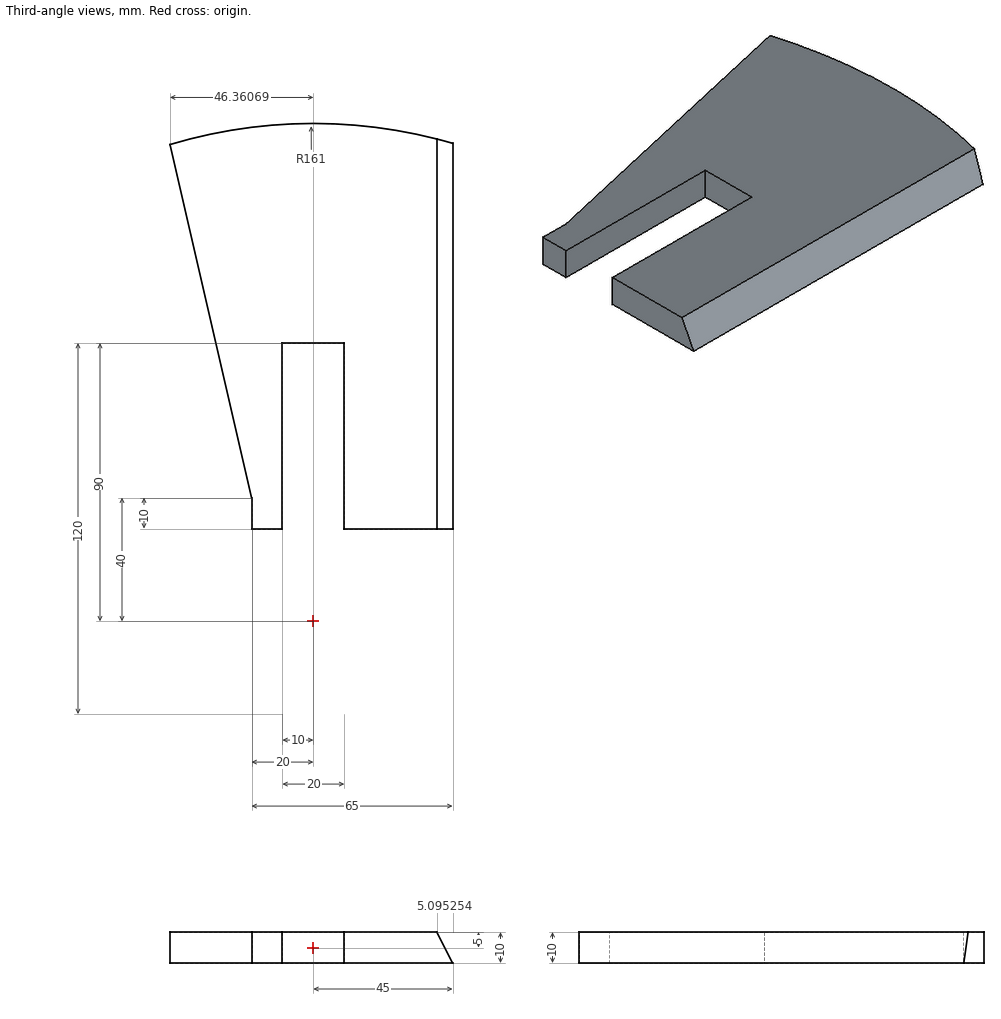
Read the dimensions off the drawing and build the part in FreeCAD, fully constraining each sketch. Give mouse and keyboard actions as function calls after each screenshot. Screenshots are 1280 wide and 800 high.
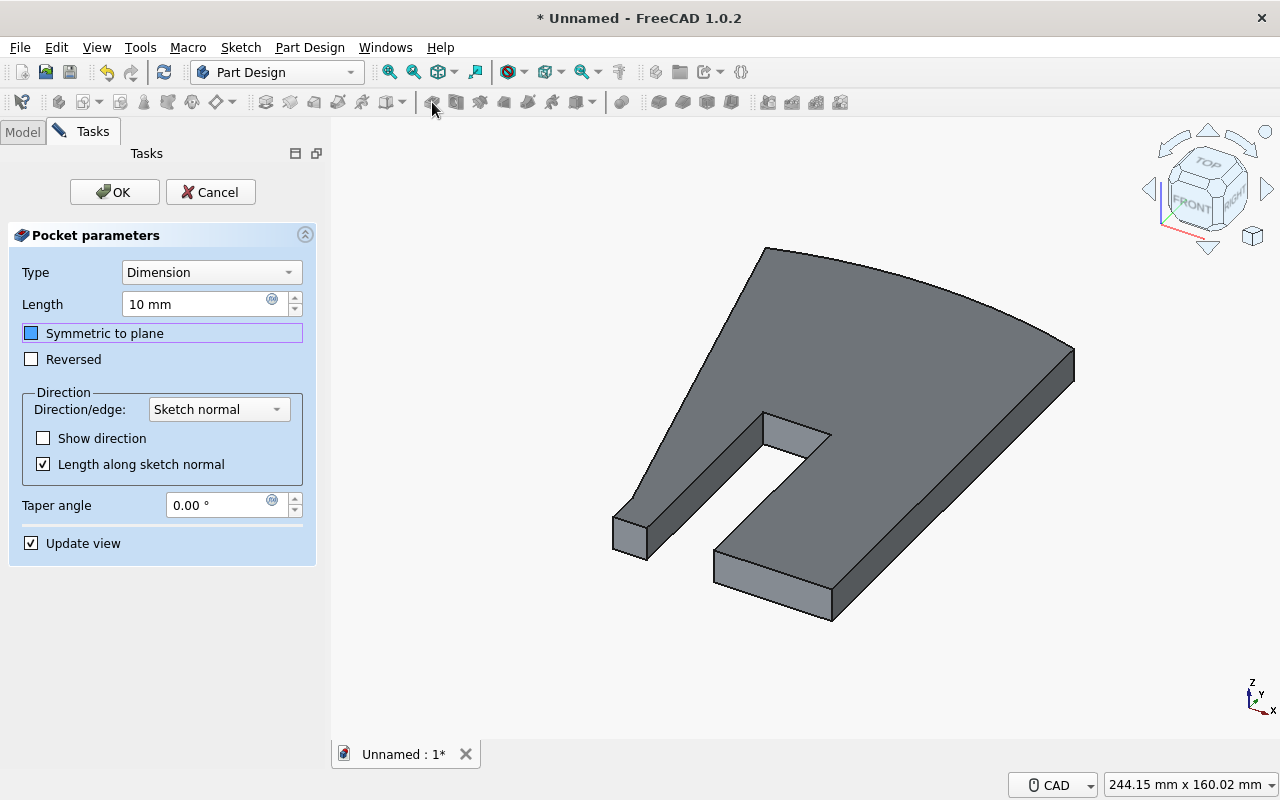
click(115, 192)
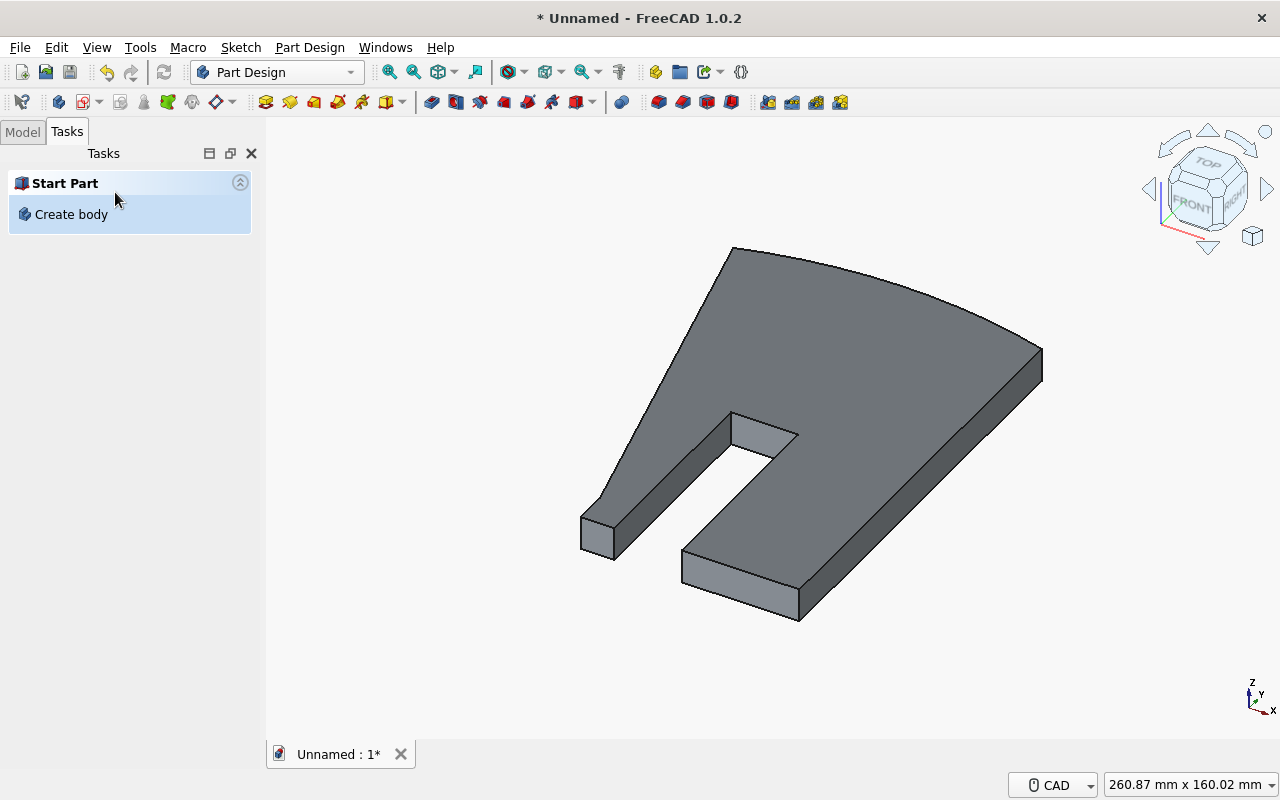
click(774, 596)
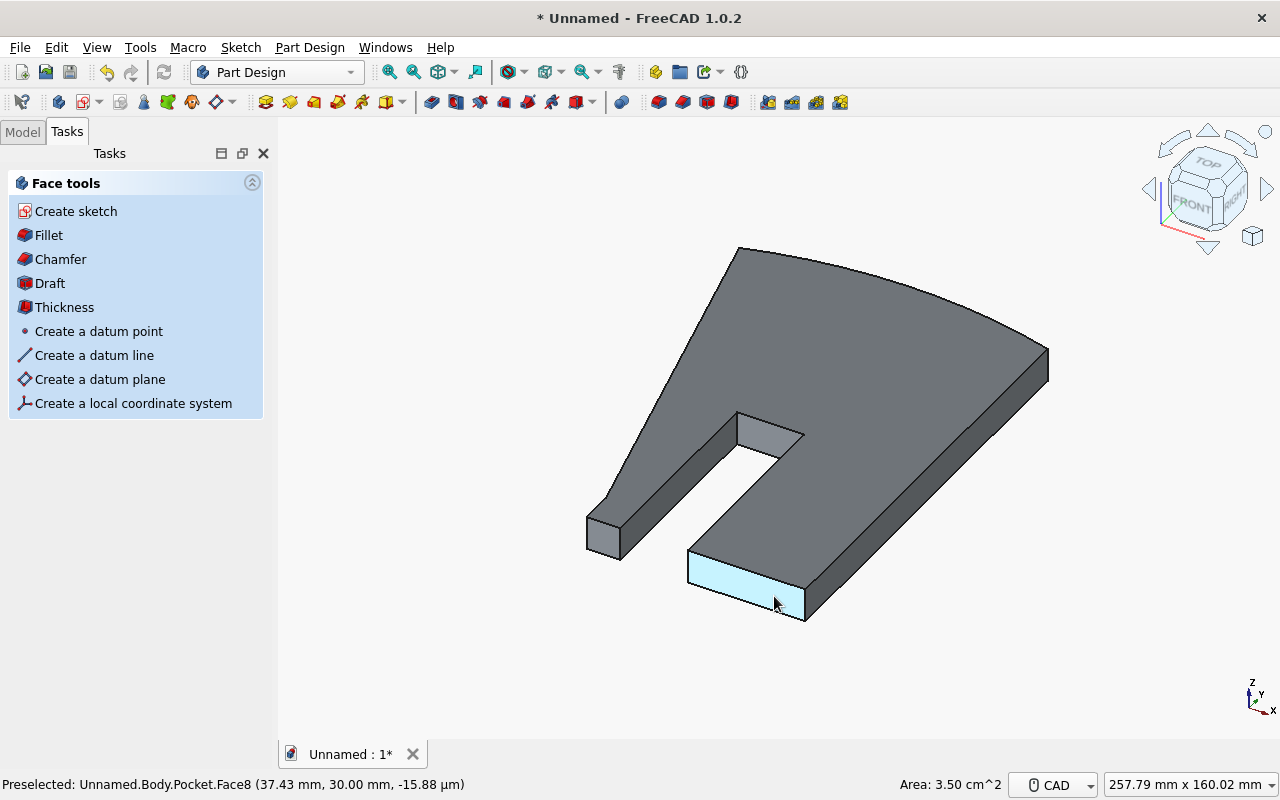
click(84, 102)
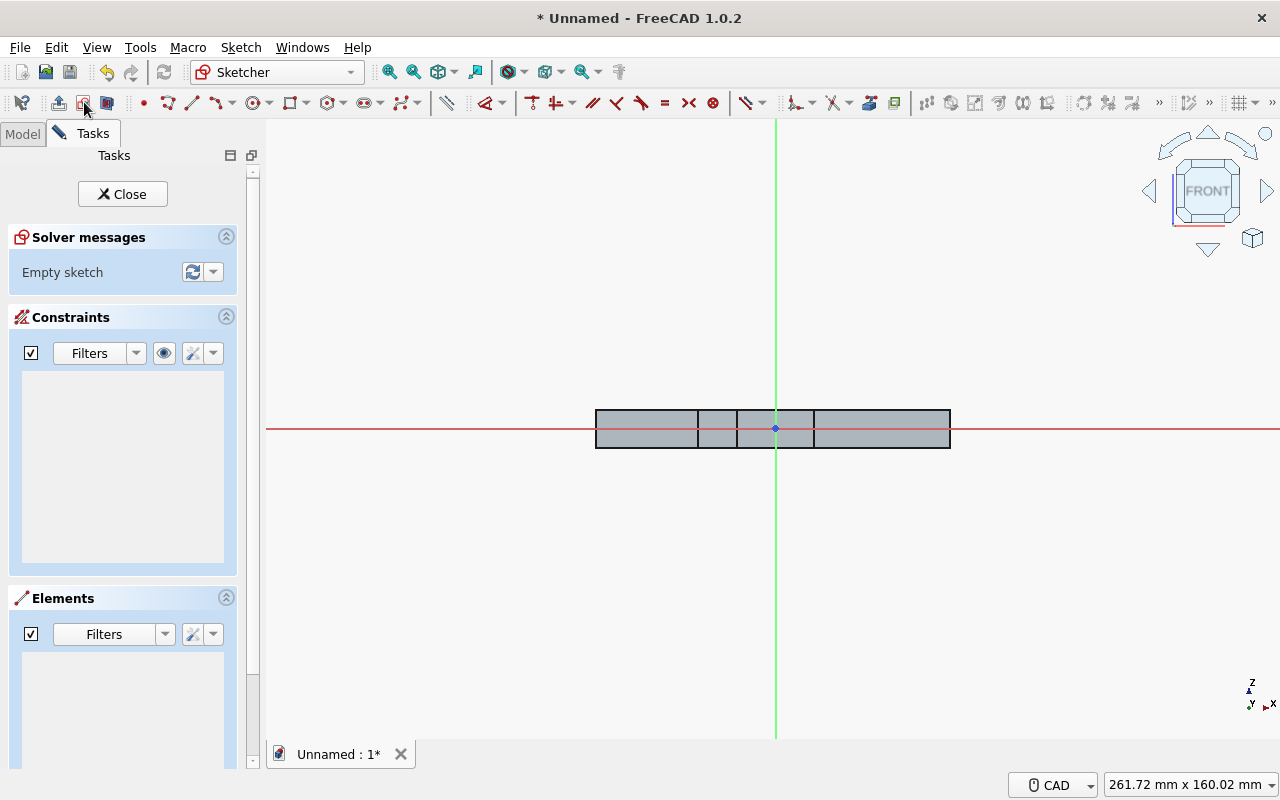
scroll(964, 429, up, 12)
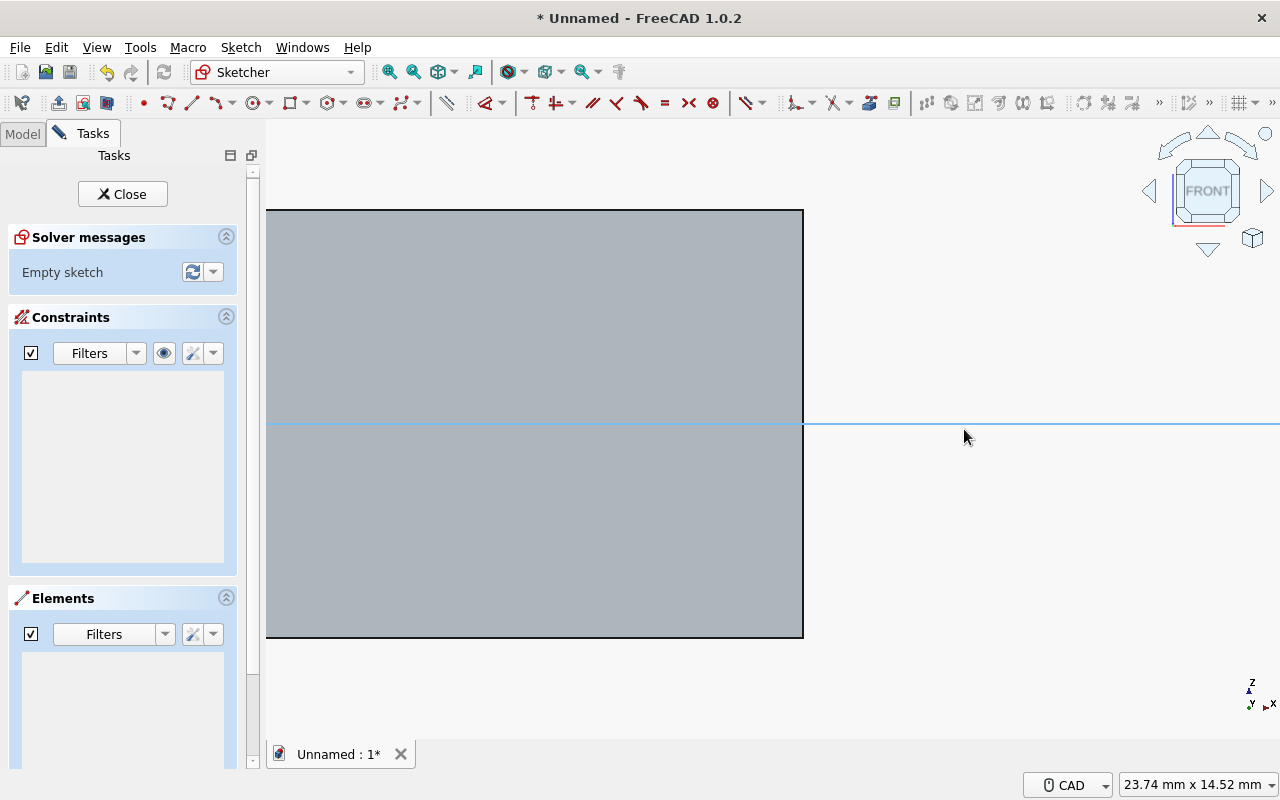
click(168, 104)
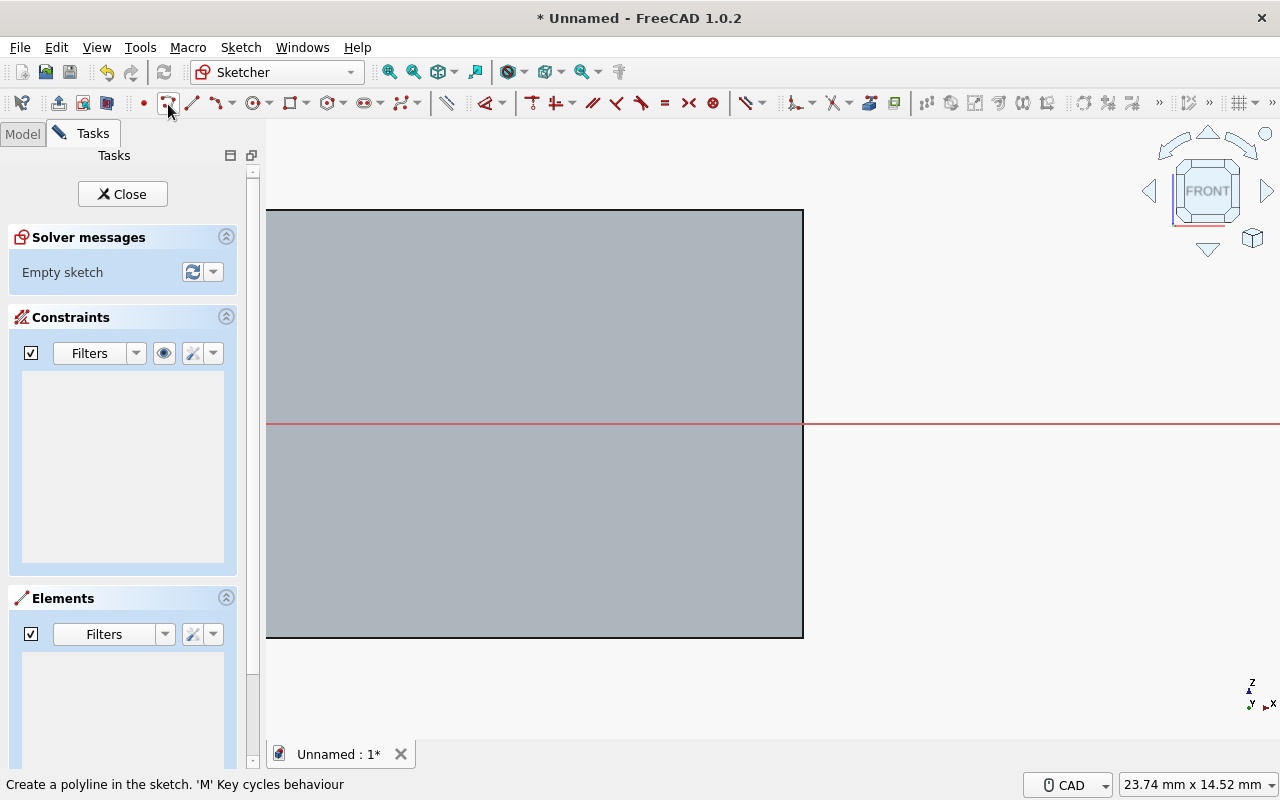
click(585, 210)
click(803, 638)
click(803, 210)
click(585, 211)
key(Escape)
key(Escape)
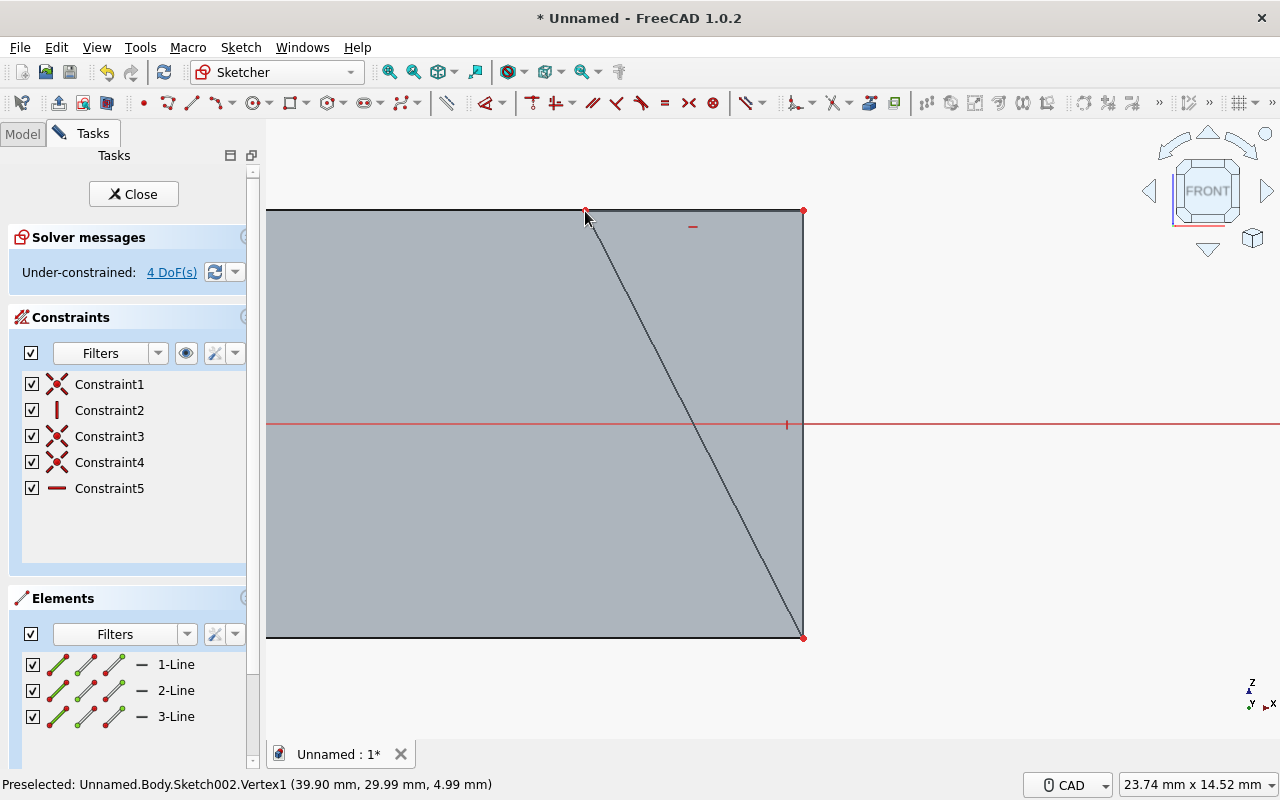
click(486, 104)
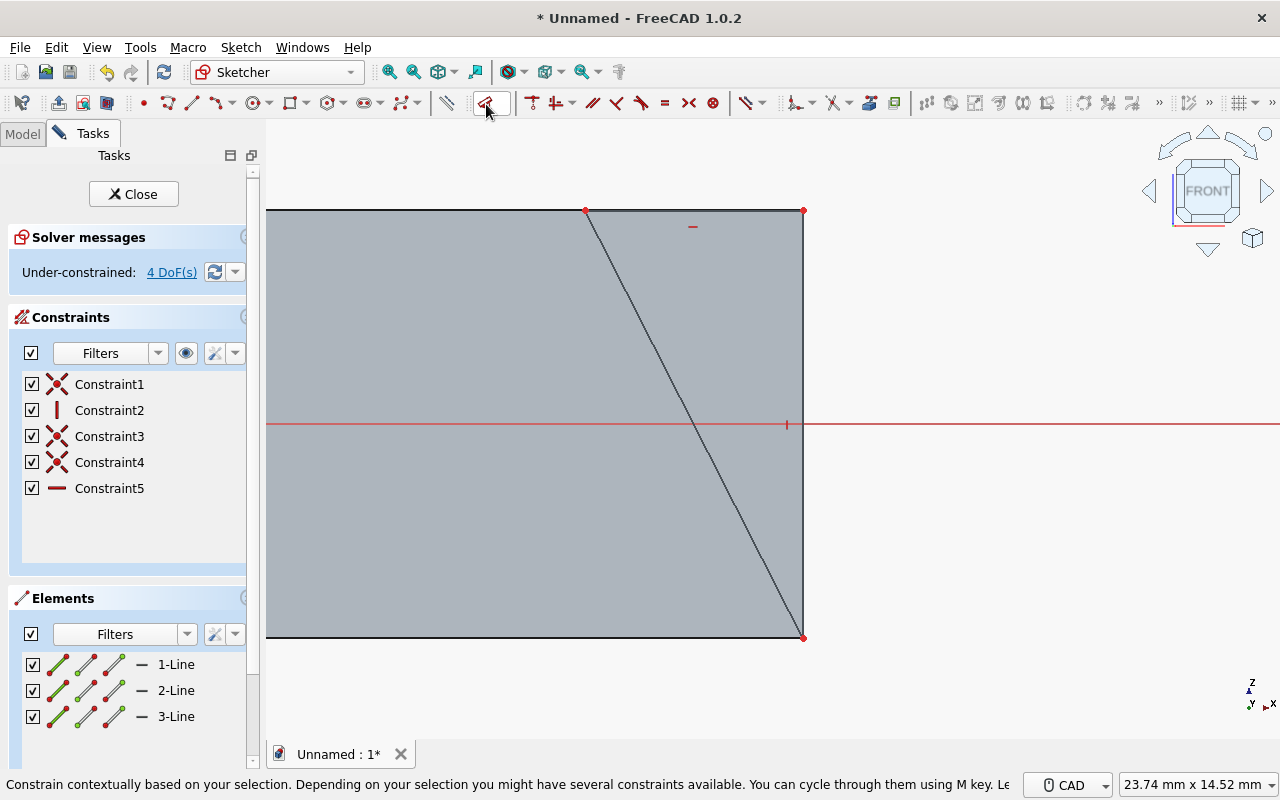
click(803, 511)
click(837, 327)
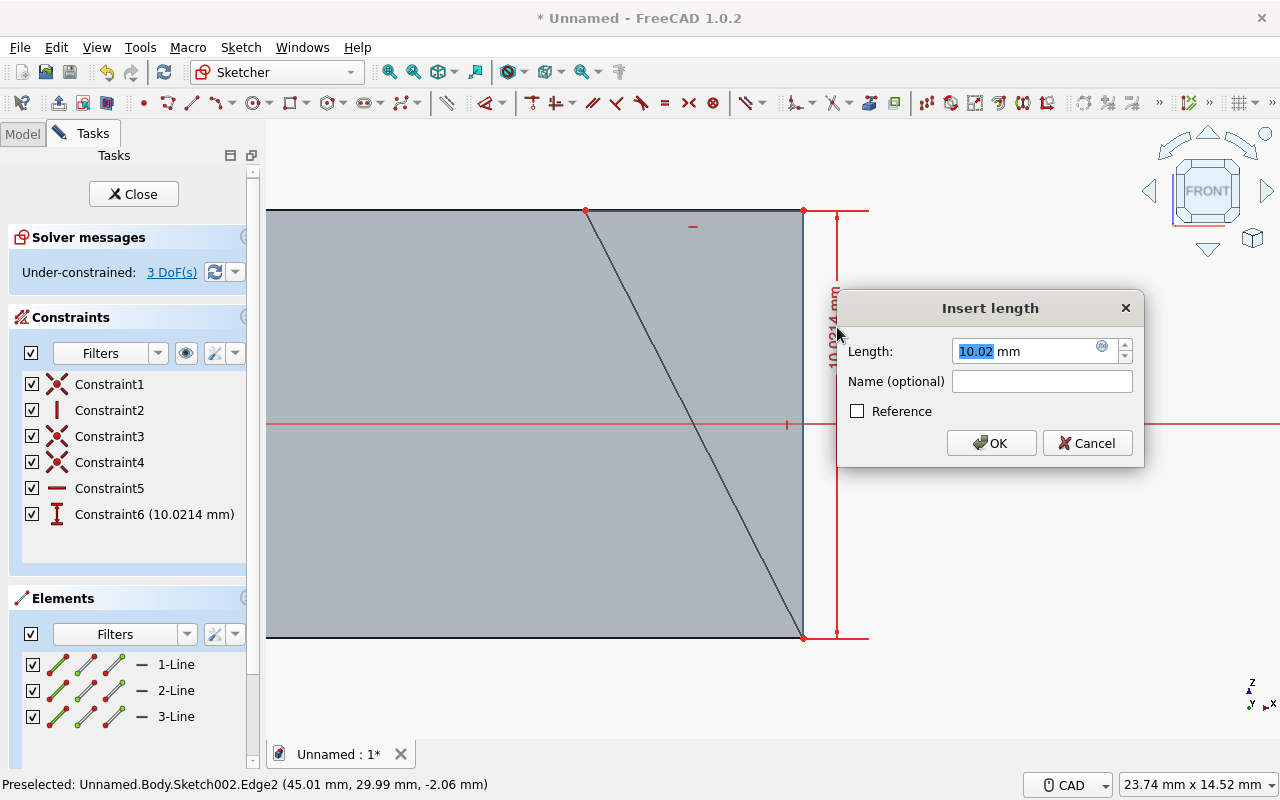
text(10)
key(Return)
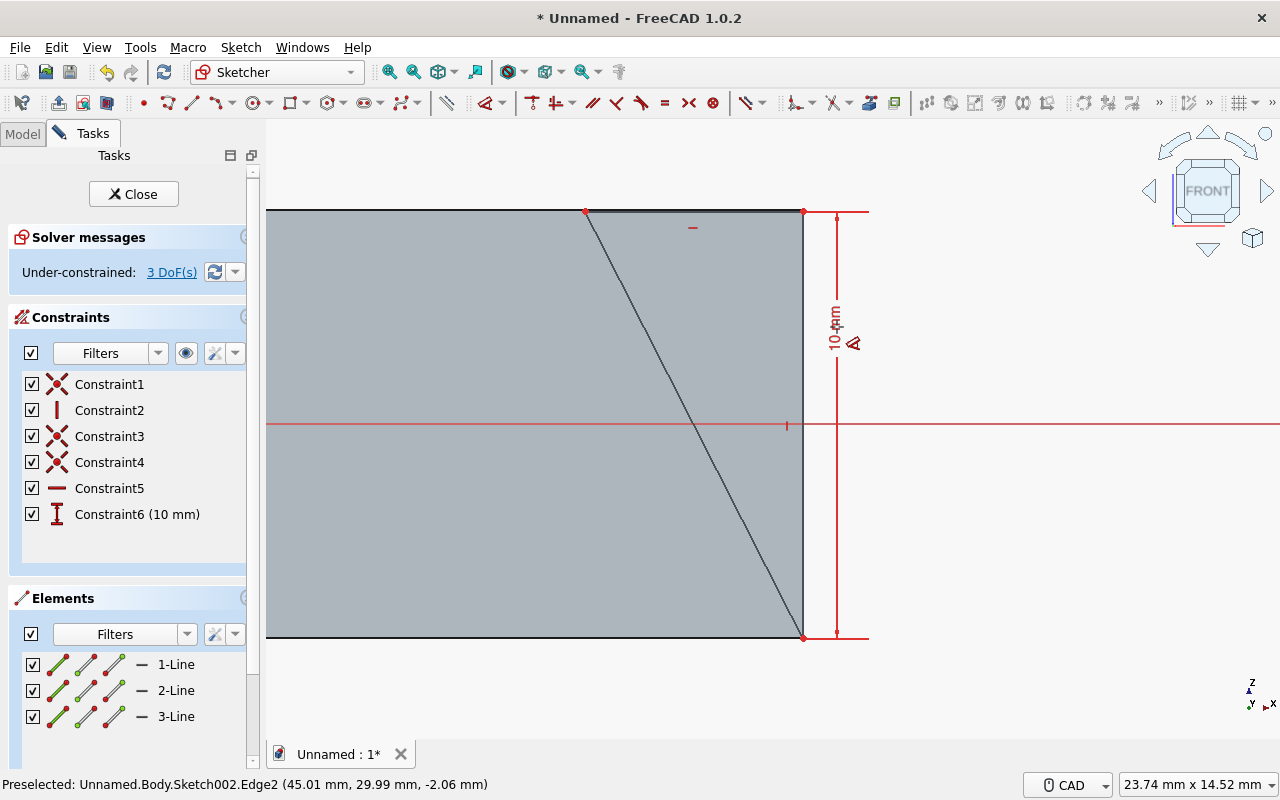
click(585, 212)
click(619, 318)